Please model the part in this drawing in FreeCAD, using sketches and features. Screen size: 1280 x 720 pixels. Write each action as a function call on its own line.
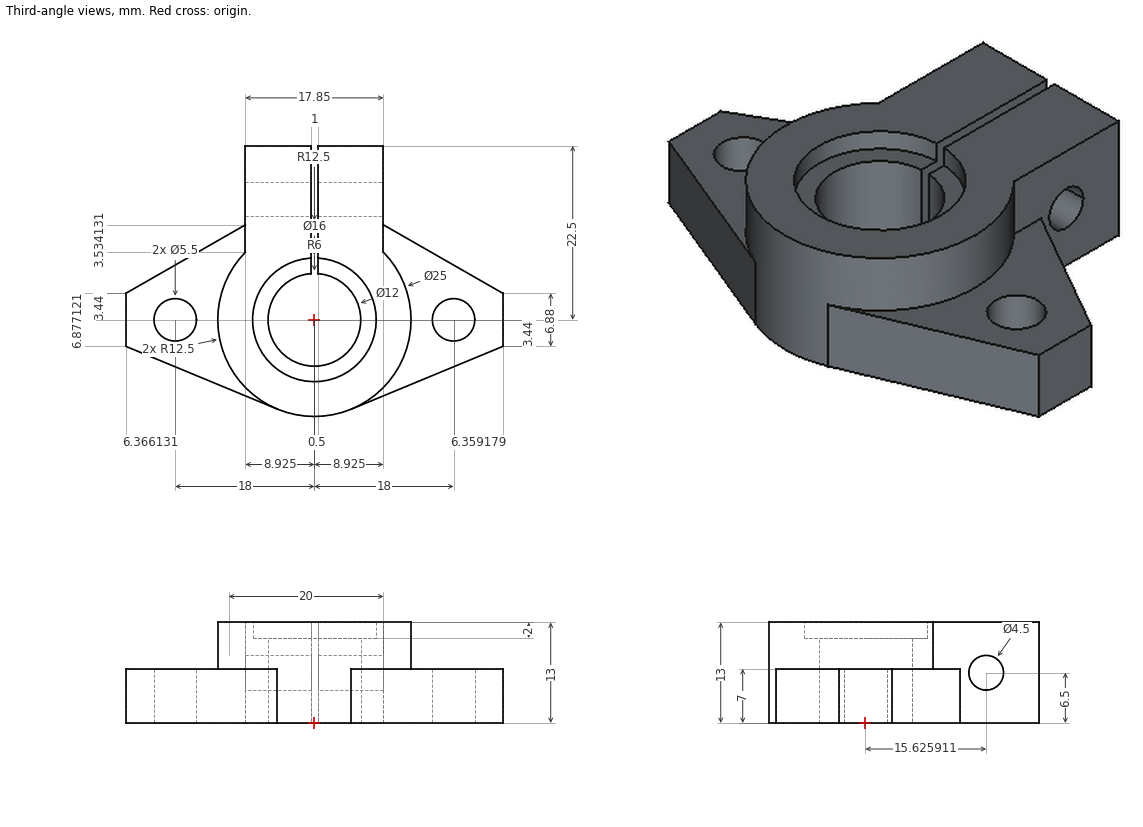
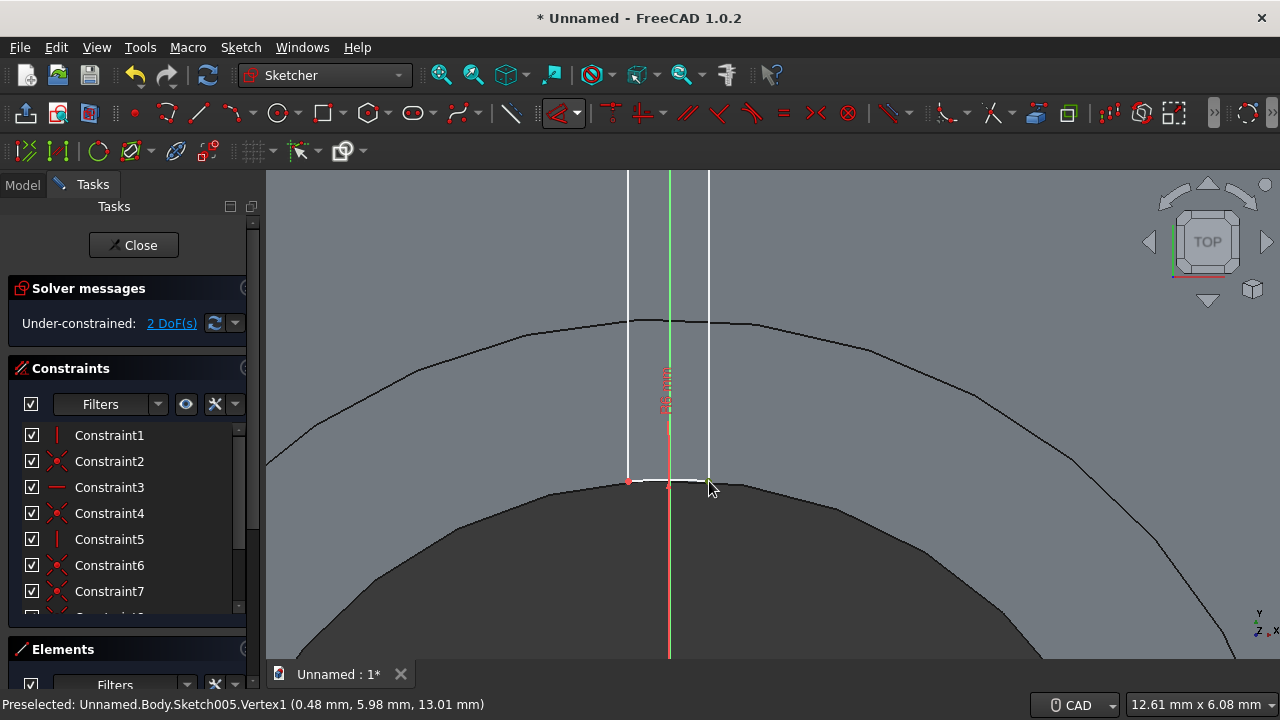
click(580, 114)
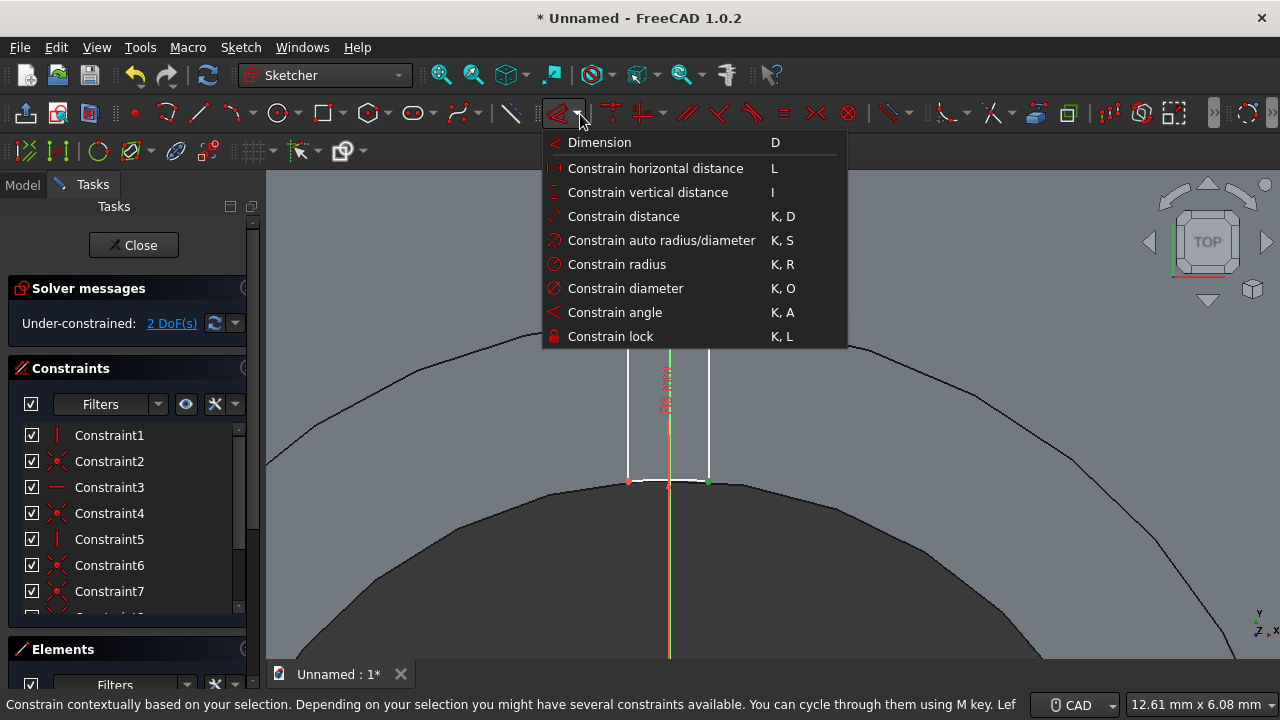
click(695, 168)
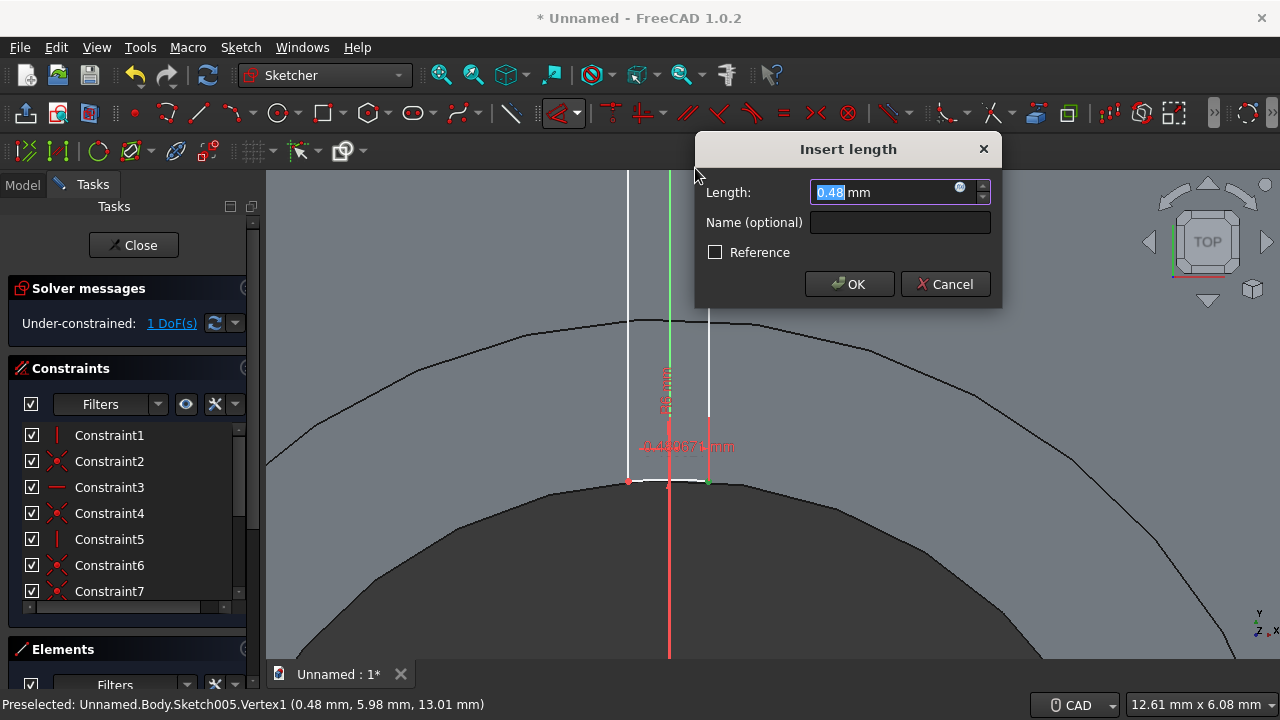
text(0.5)
key(Return)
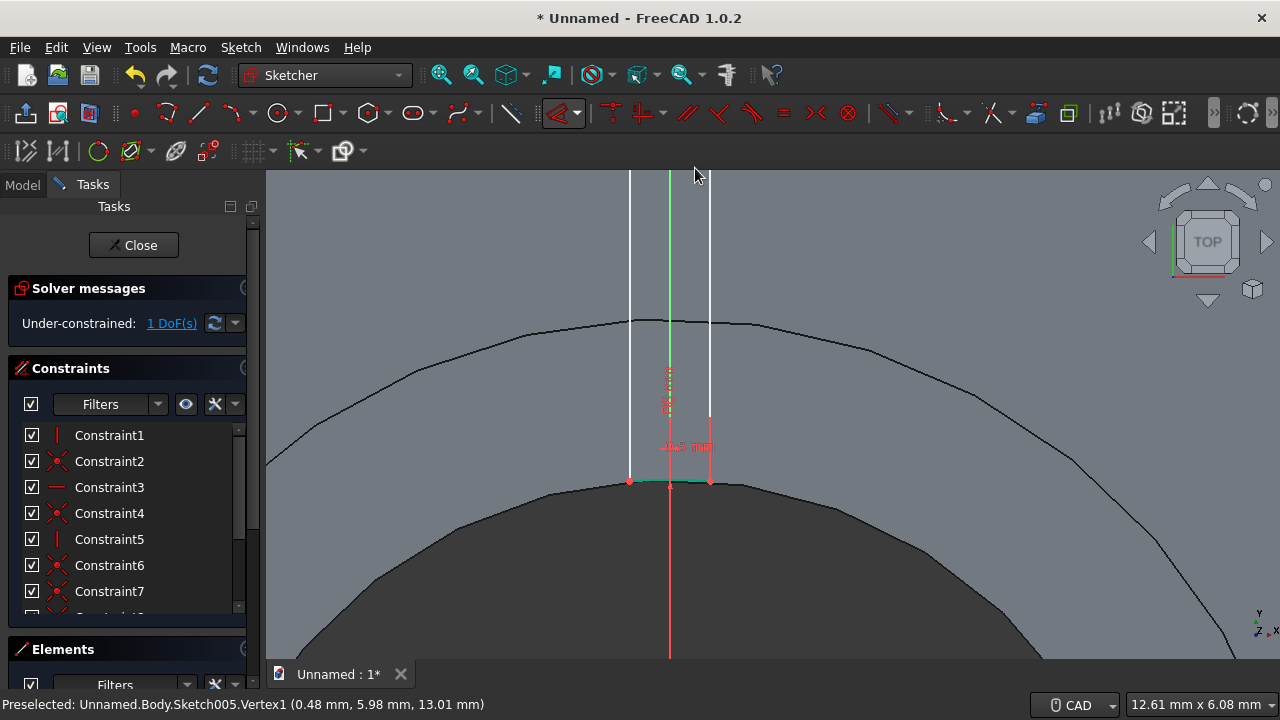
scroll(711, 485, down, 9)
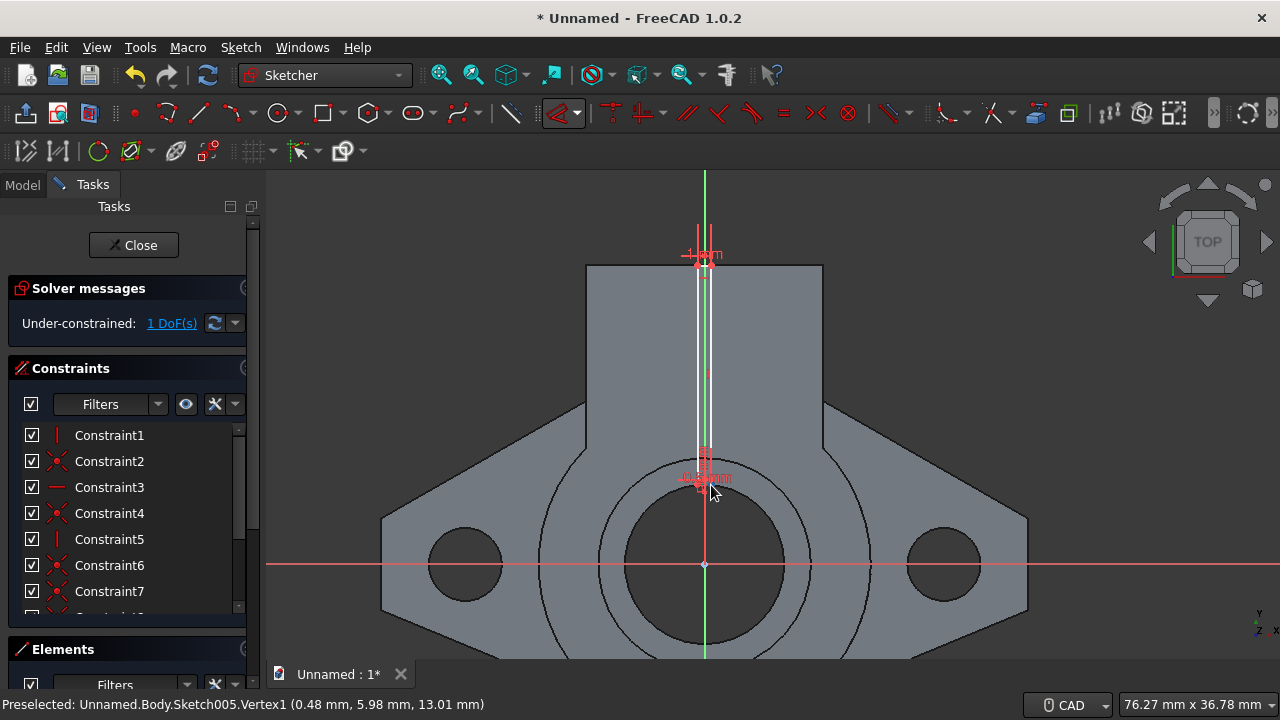
click(711, 266)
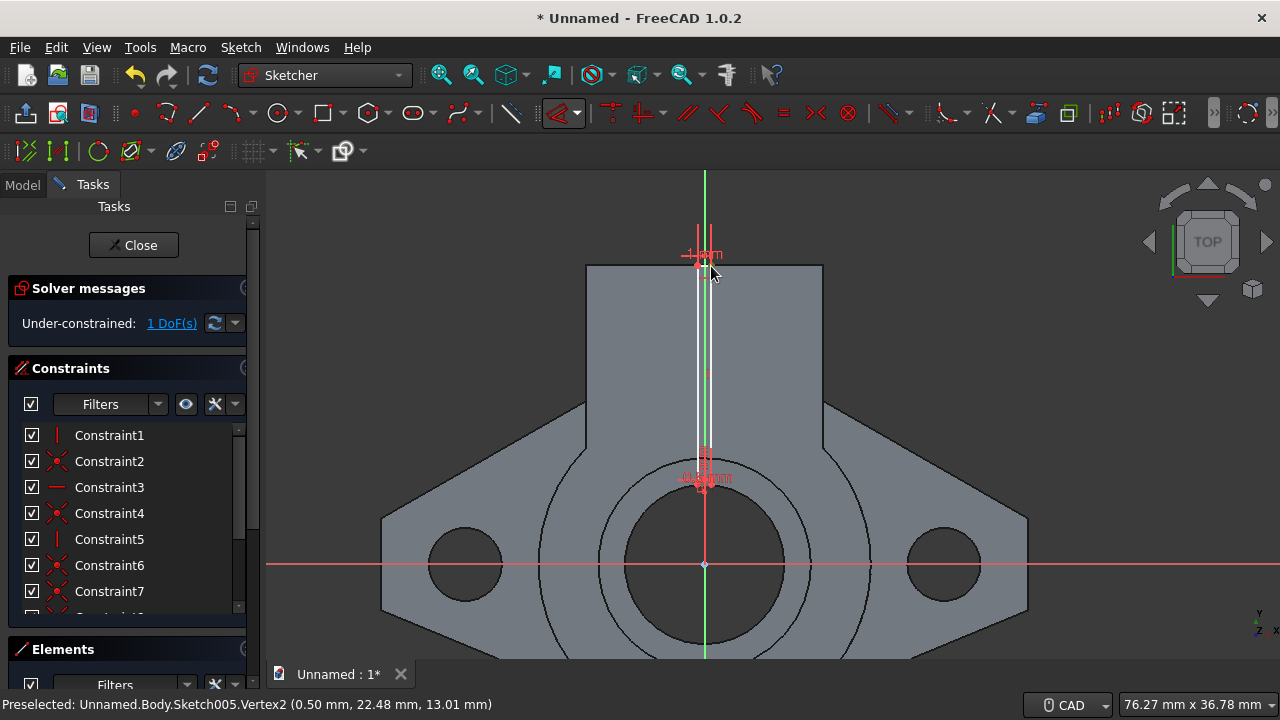
click(580, 114)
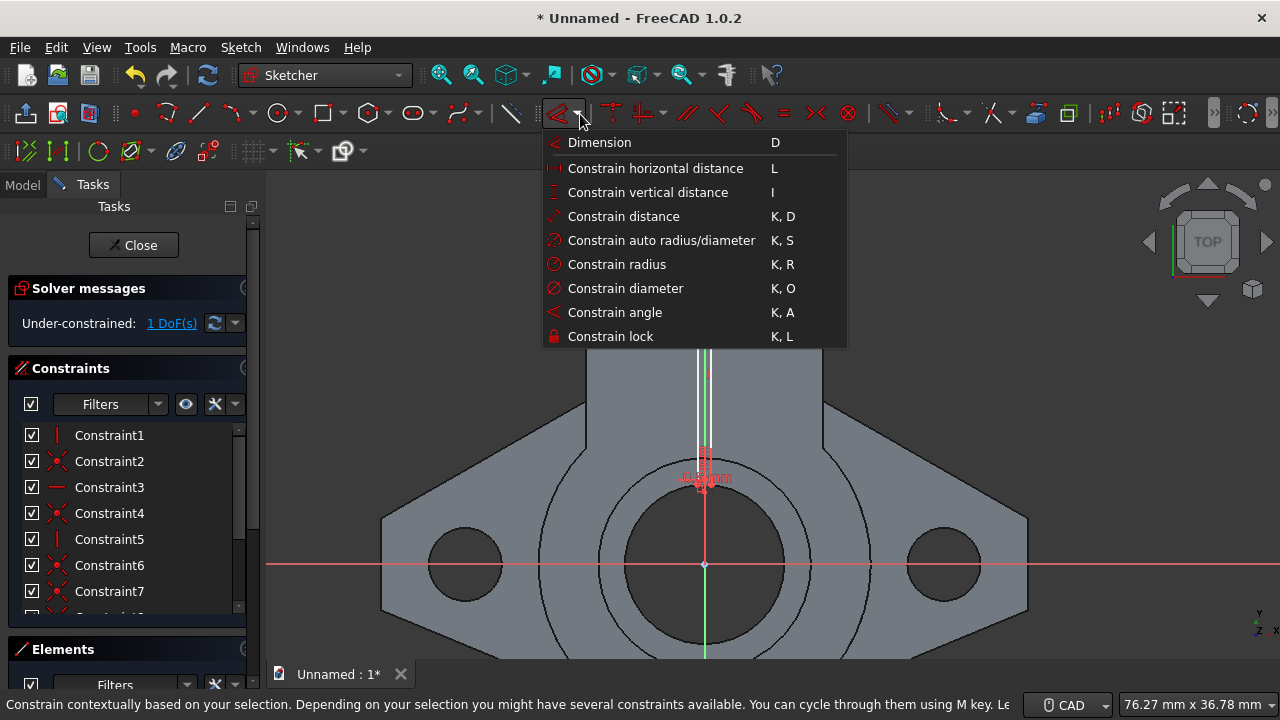
click(695, 192)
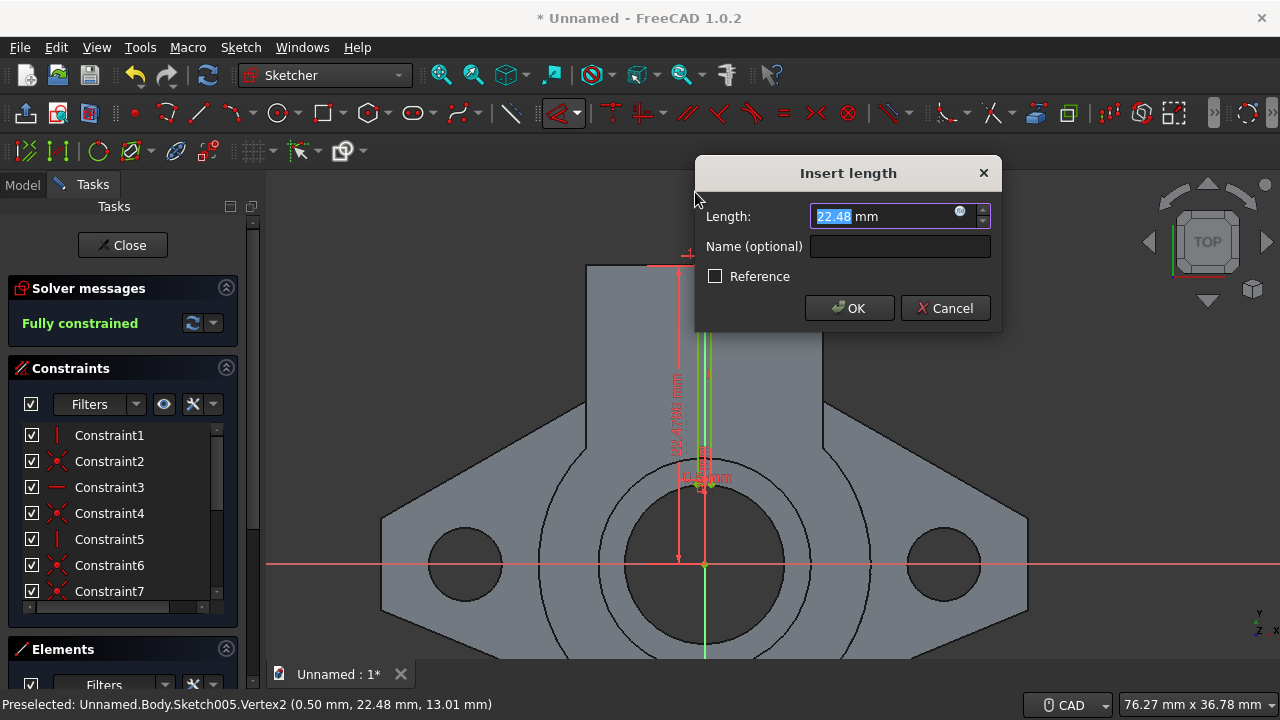
text(22.5)
key(Return)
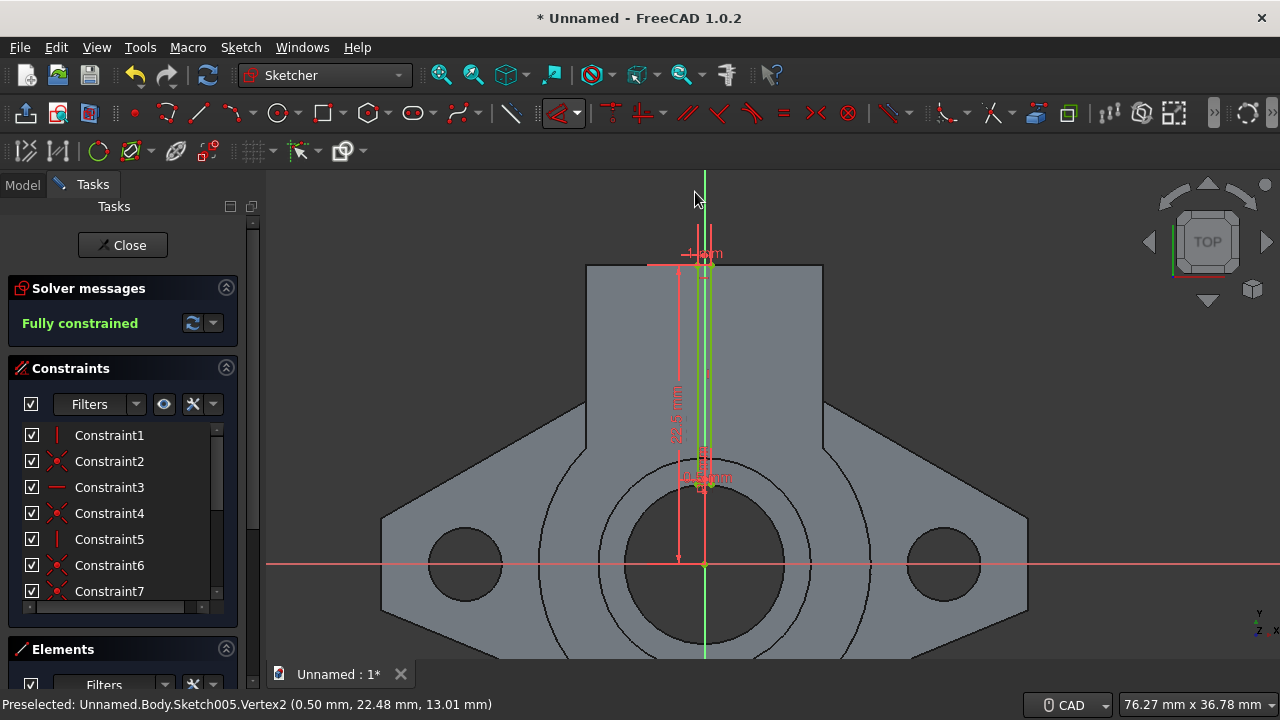
click(123, 245)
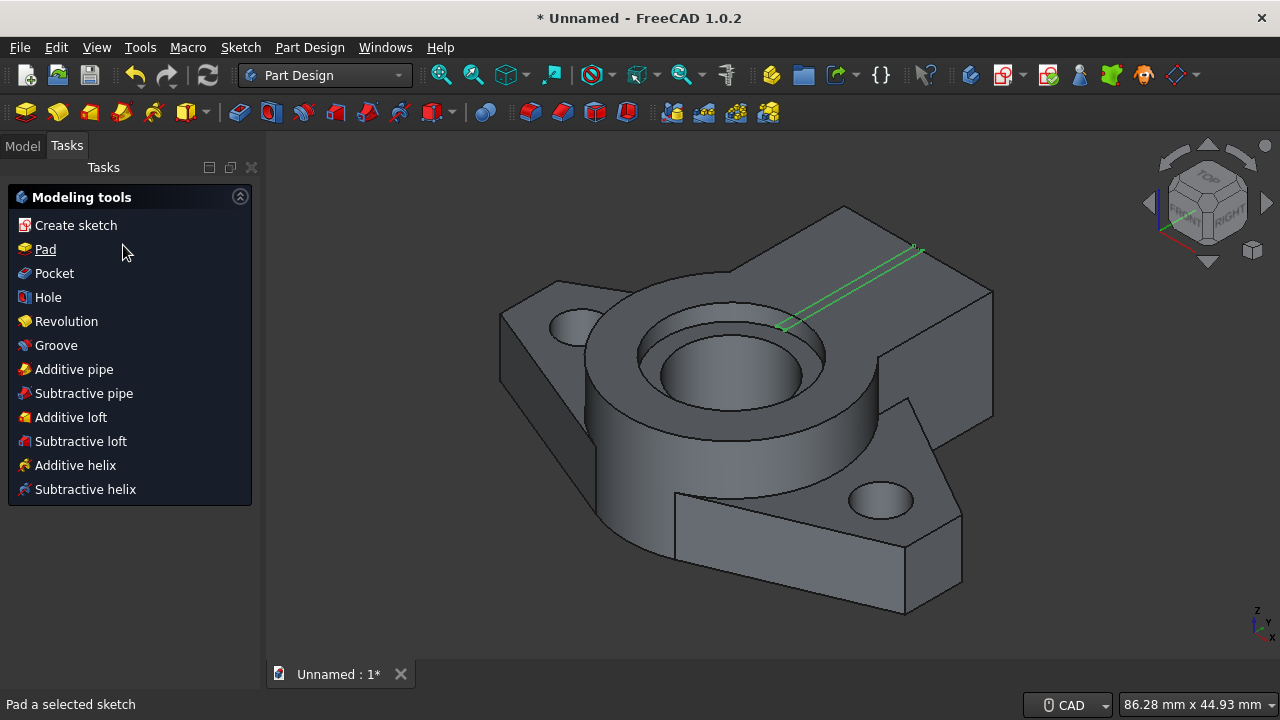
click(240, 112)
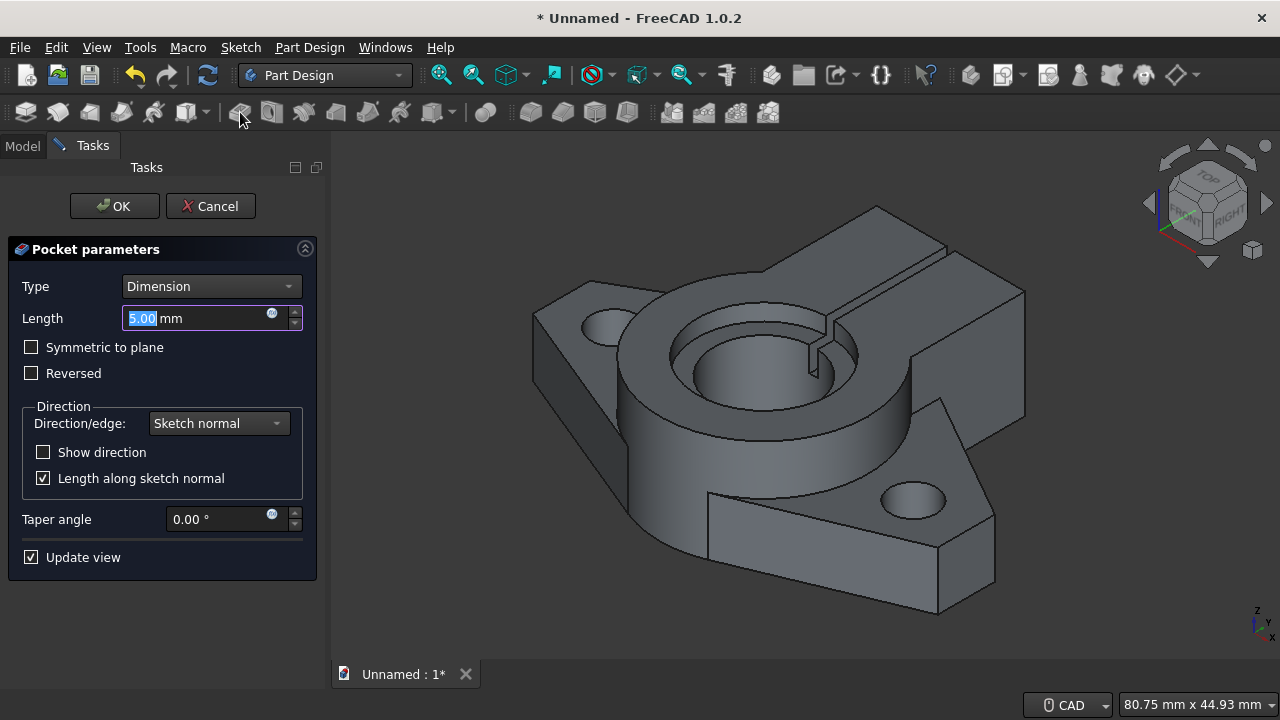
click(212, 286)